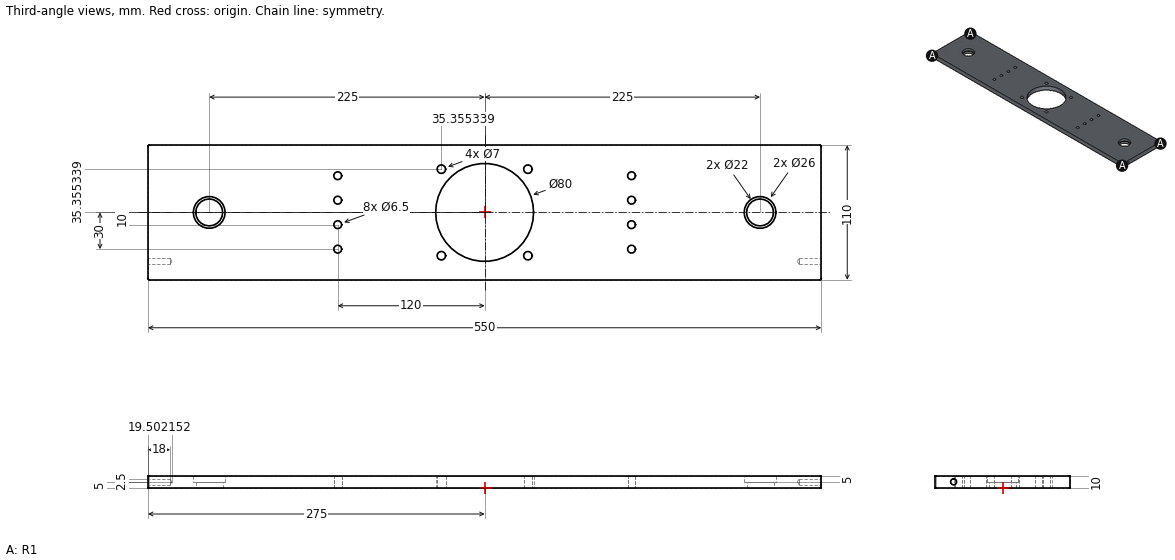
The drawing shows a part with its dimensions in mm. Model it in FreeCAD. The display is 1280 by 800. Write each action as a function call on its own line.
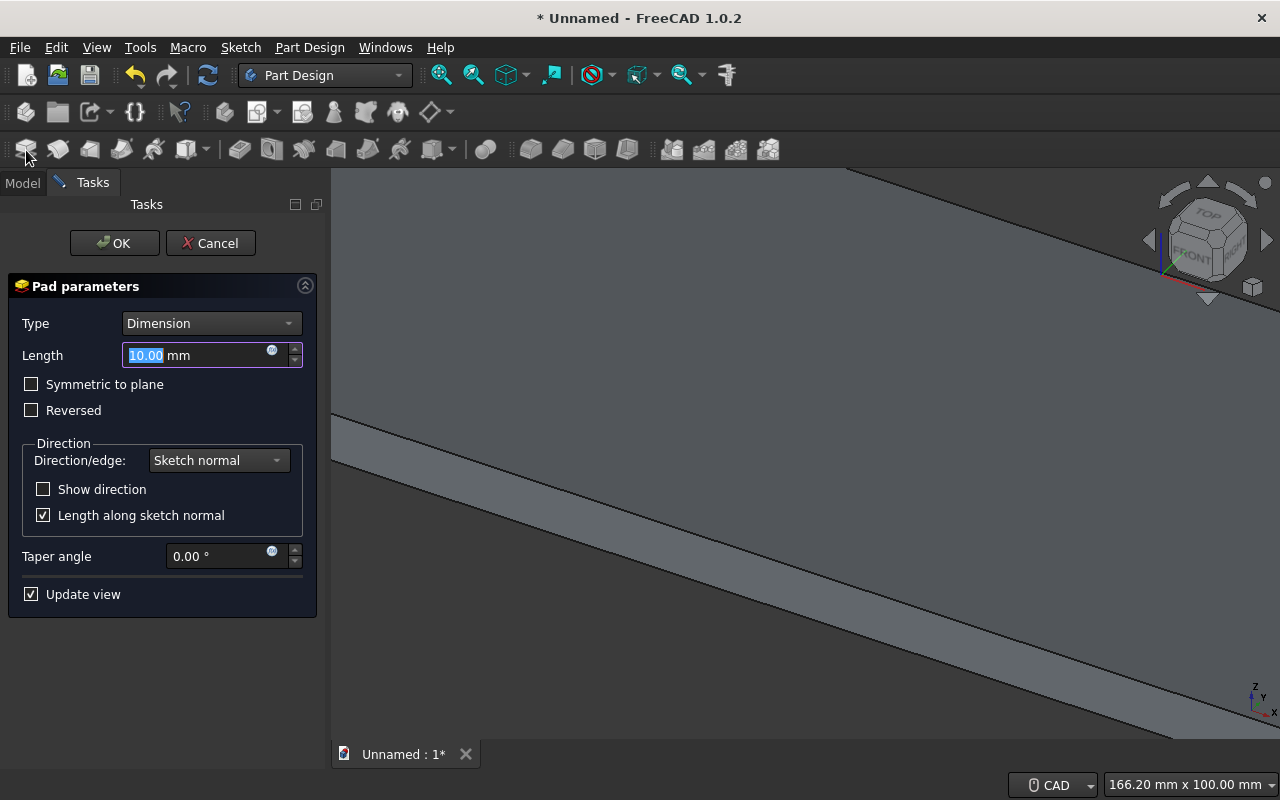
text(10)
key(Tab)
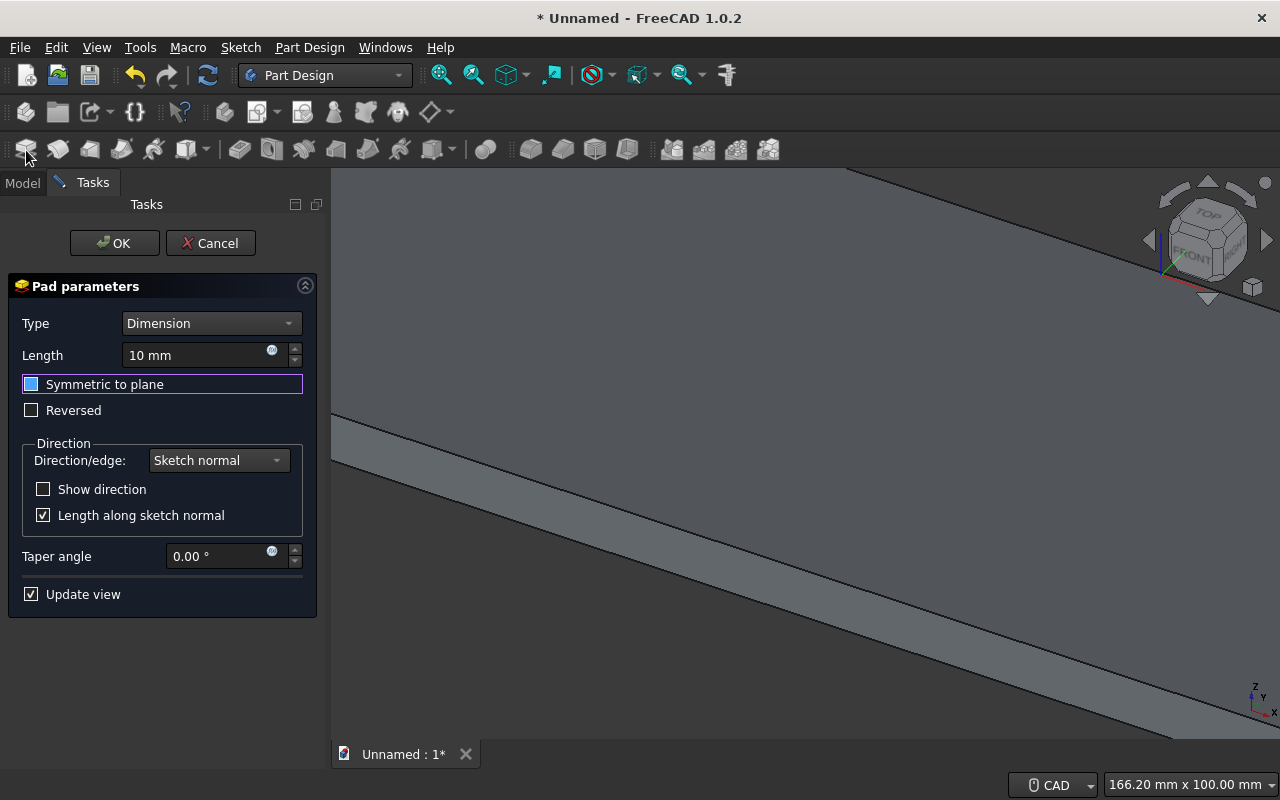
click(115, 243)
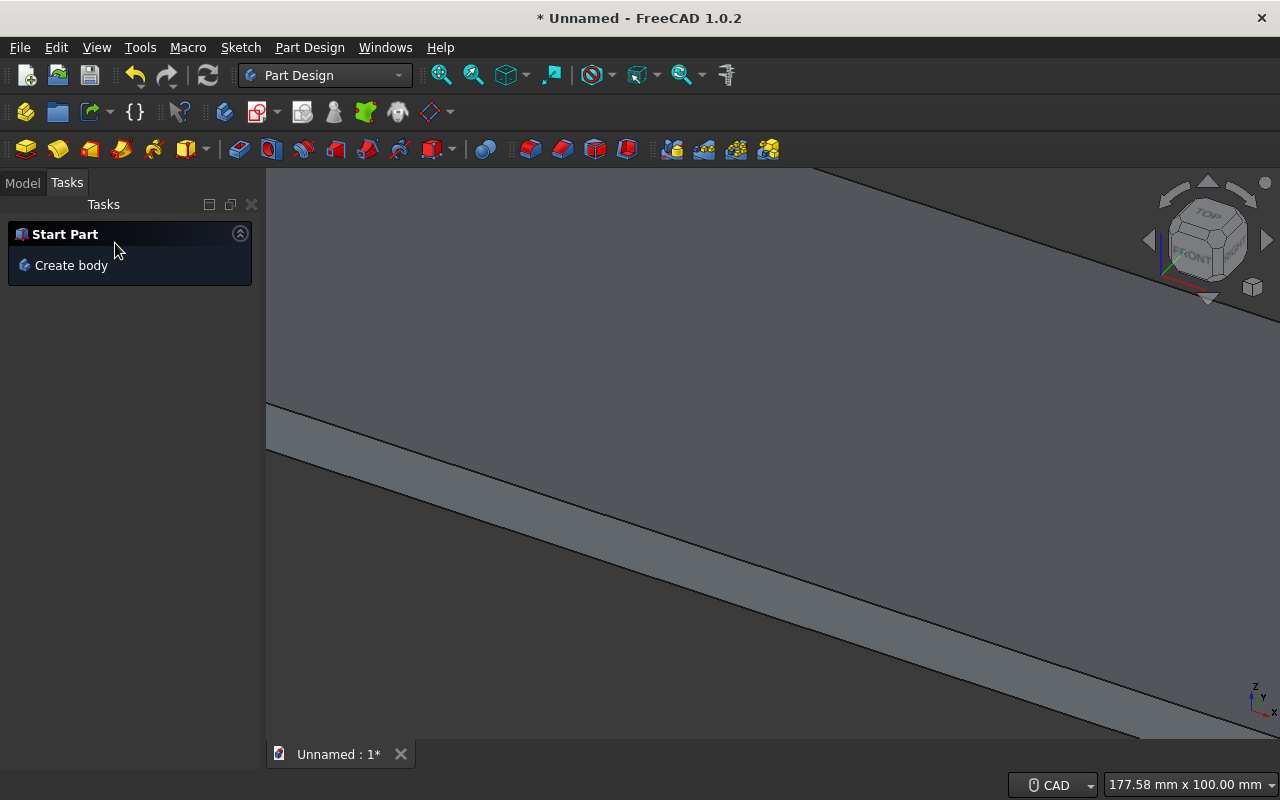
click(442, 76)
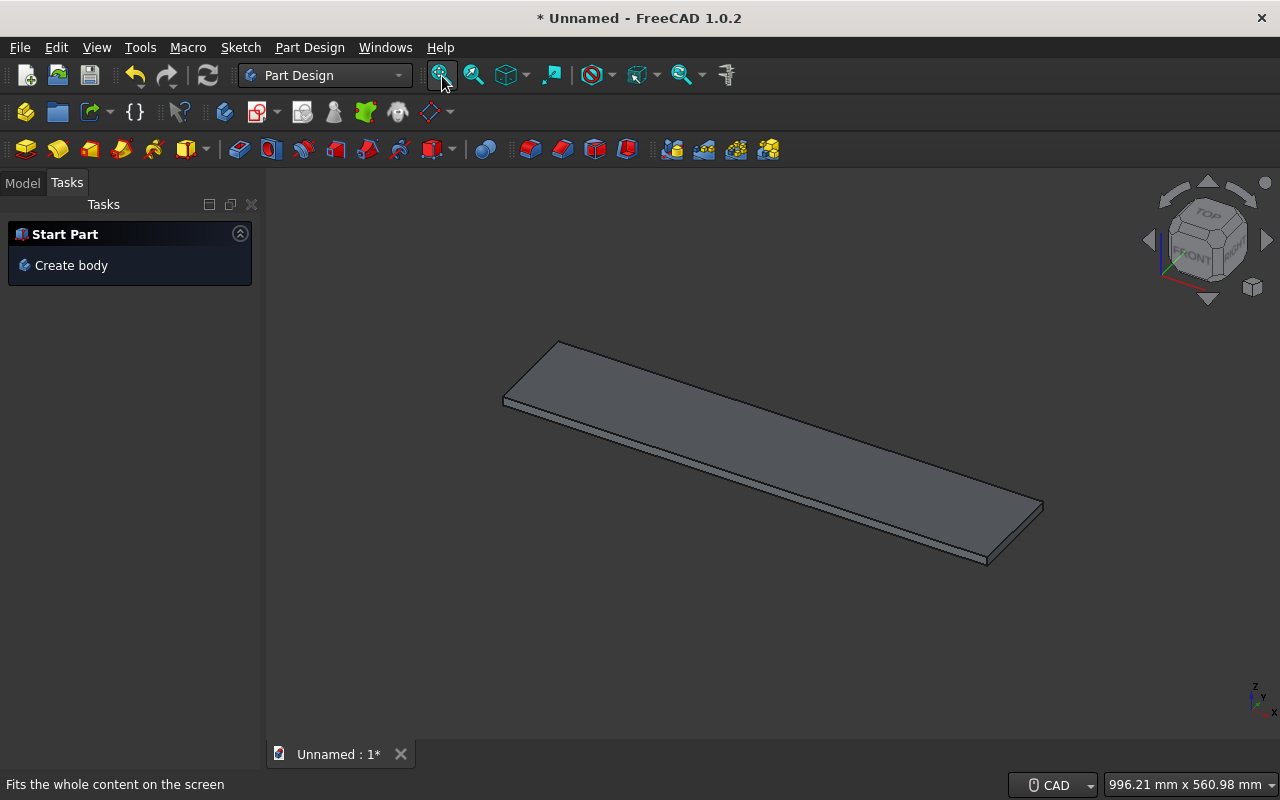
click(912, 494)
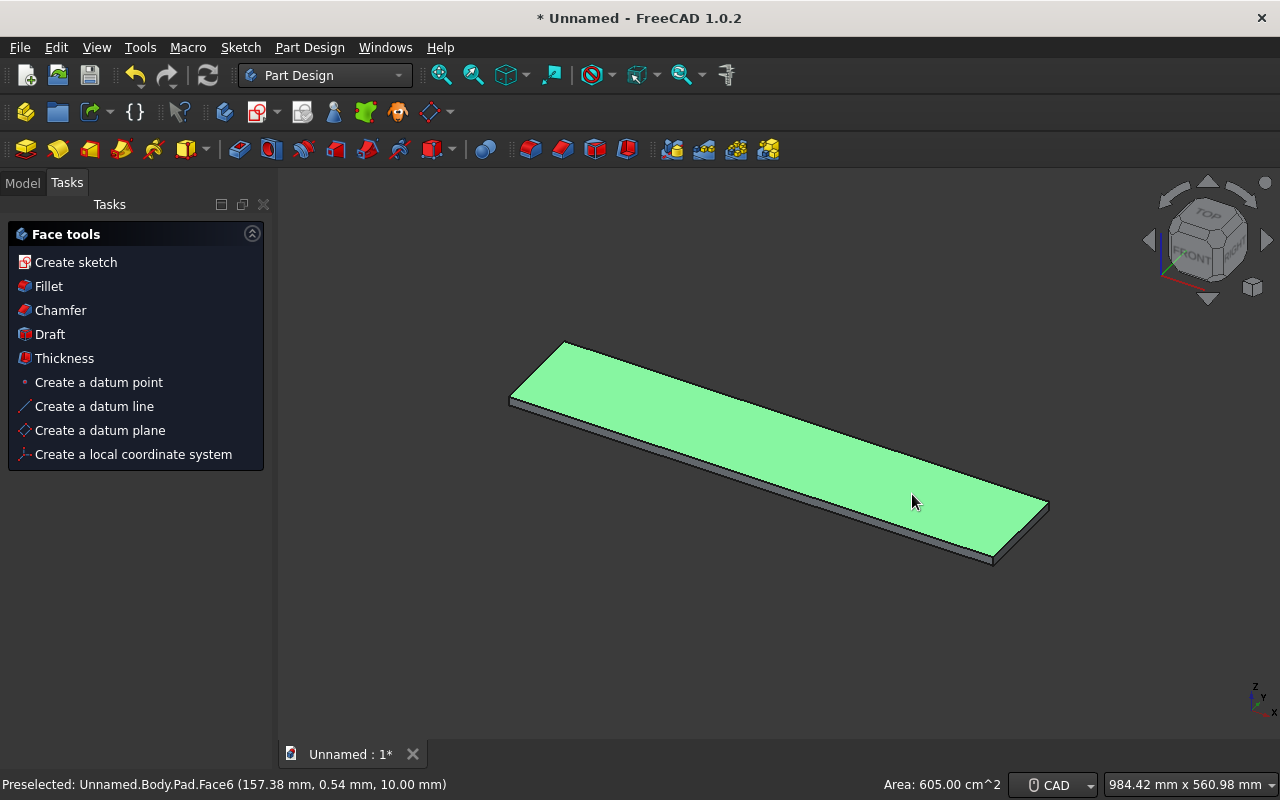
click(258, 112)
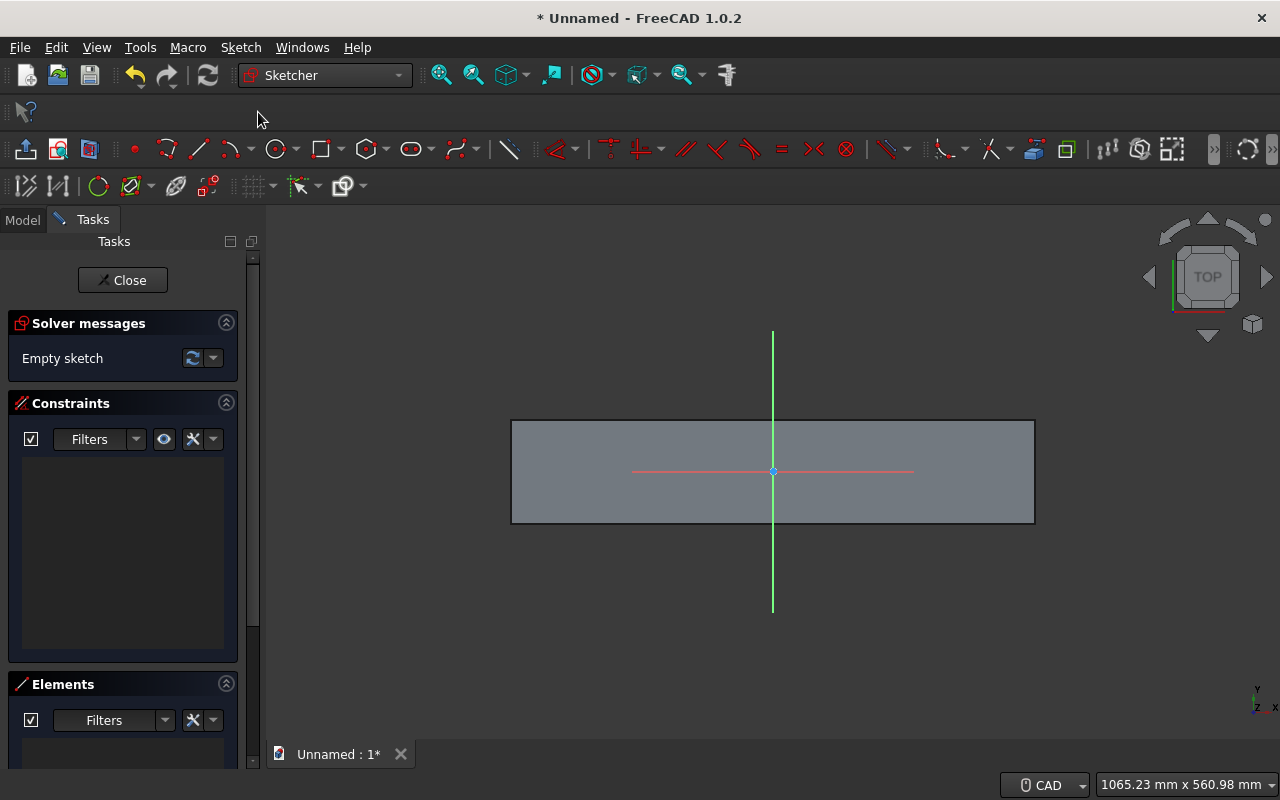
key(g)
key(c)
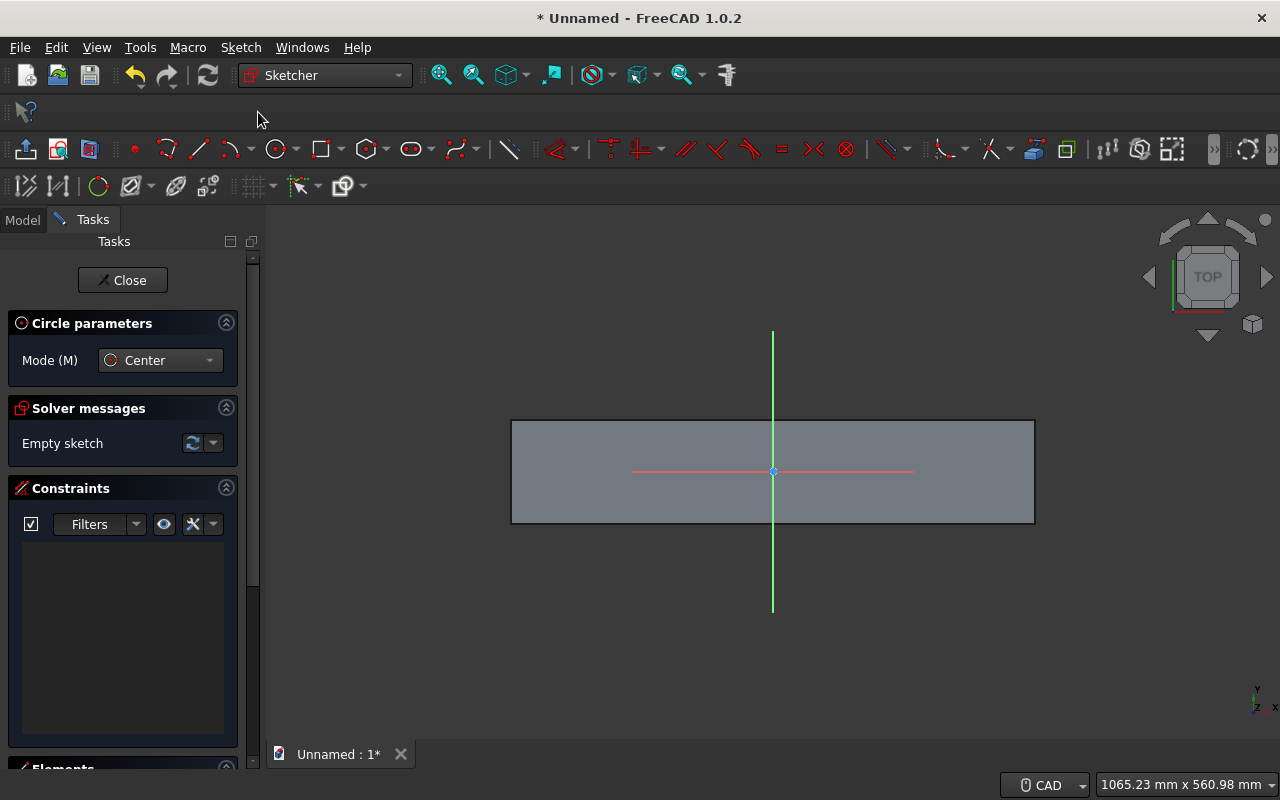
scroll(987, 472, up, 4)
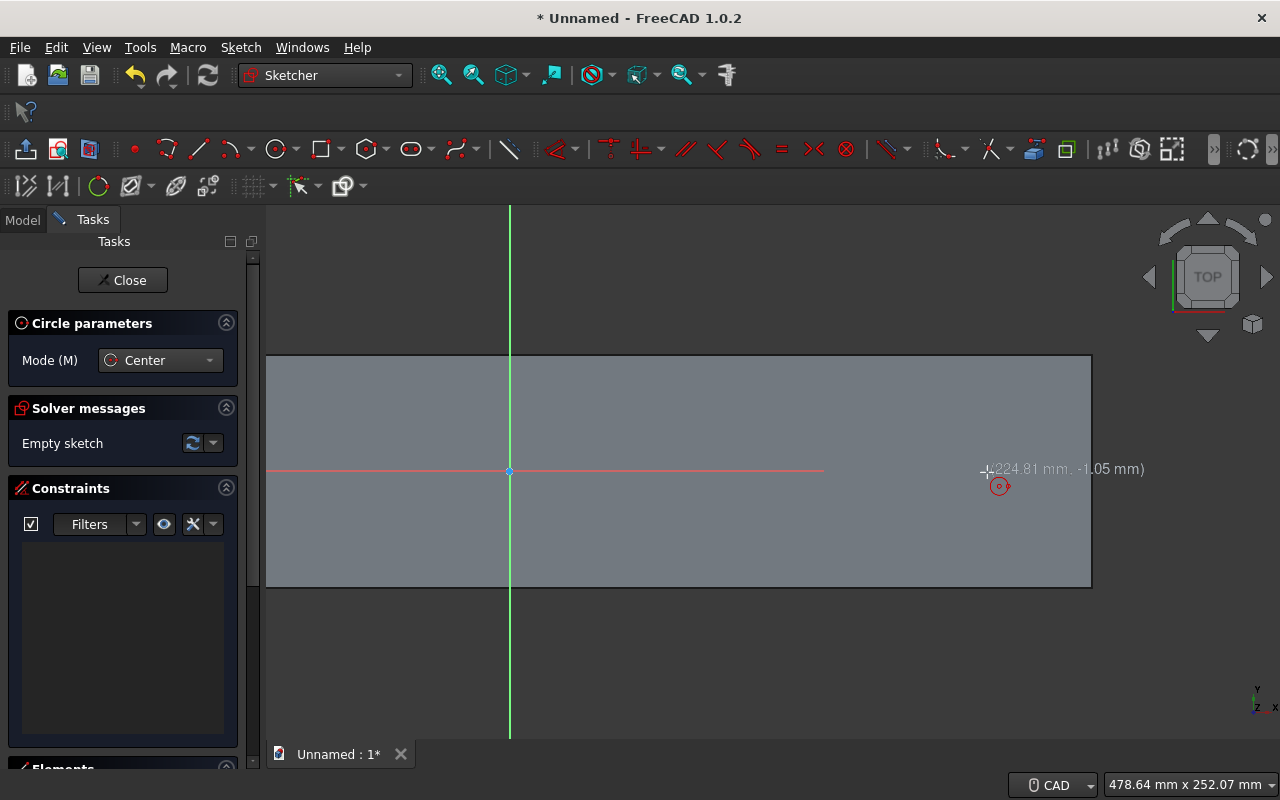
click(987, 471)
move(1006, 452)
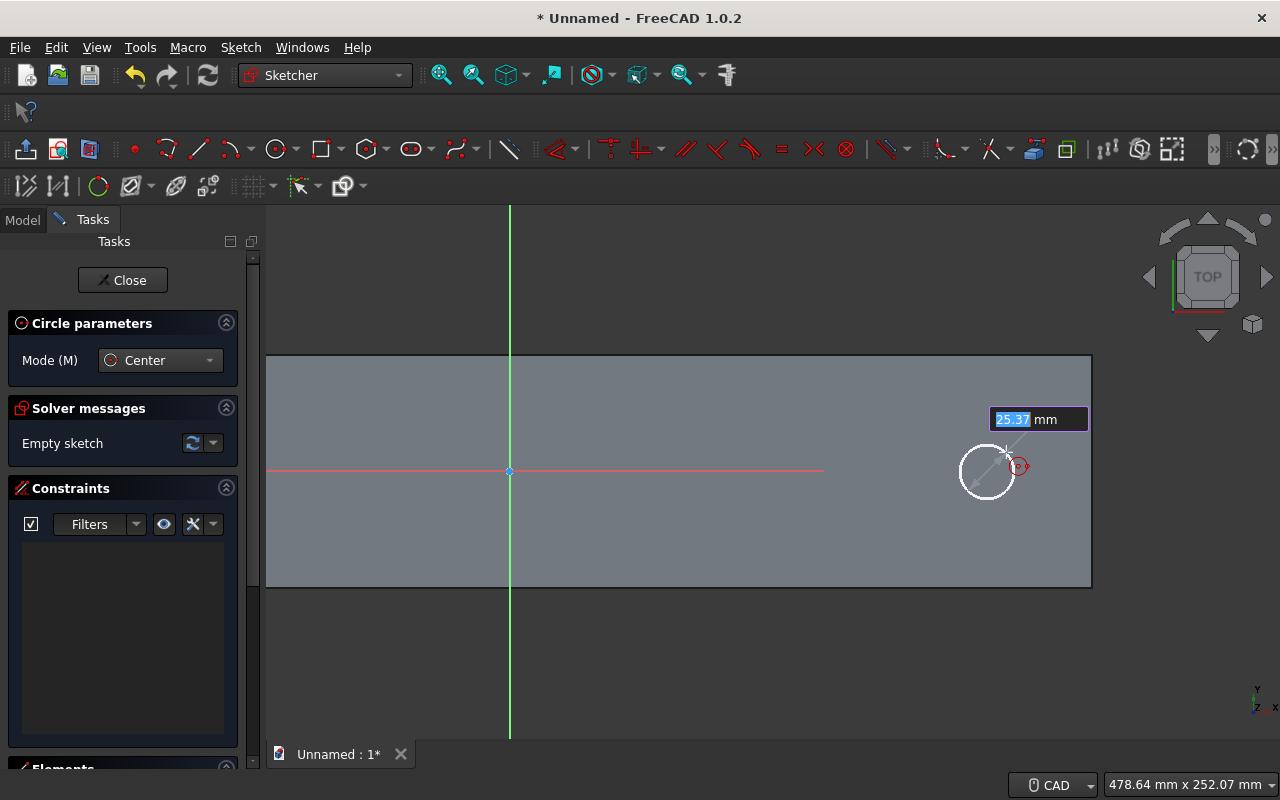
text(26)
key(Return)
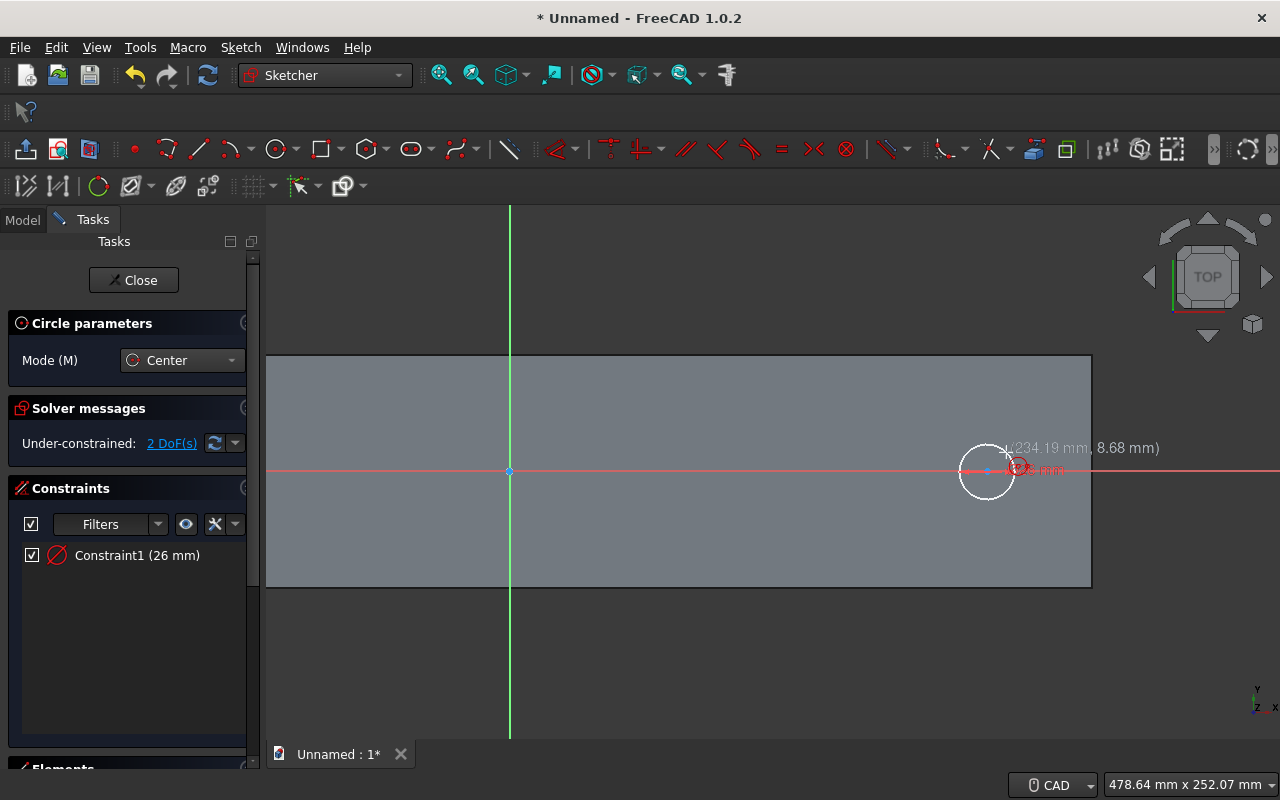
scroll(941, 473, down, 3)